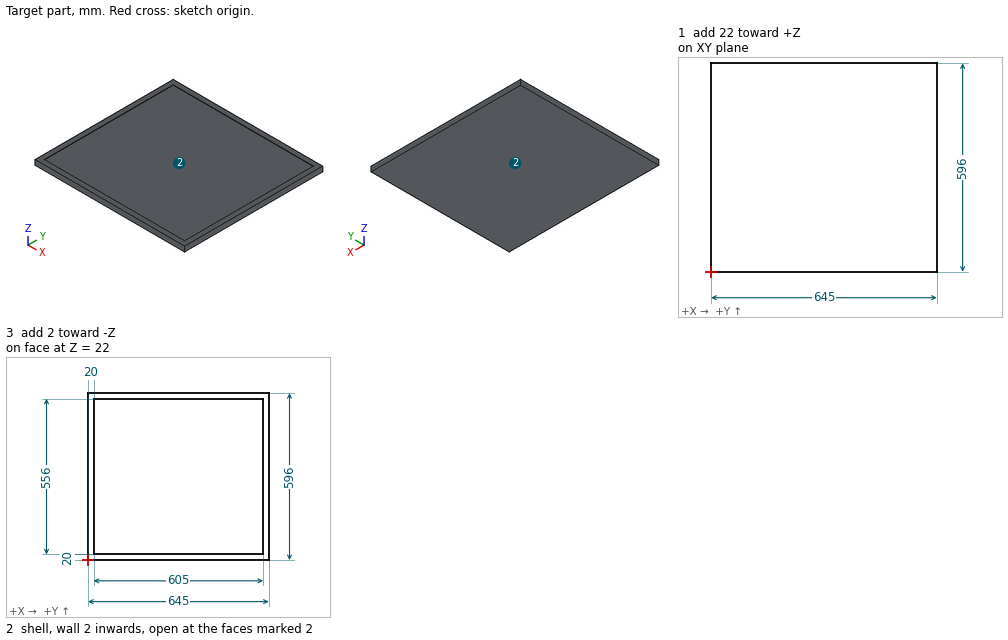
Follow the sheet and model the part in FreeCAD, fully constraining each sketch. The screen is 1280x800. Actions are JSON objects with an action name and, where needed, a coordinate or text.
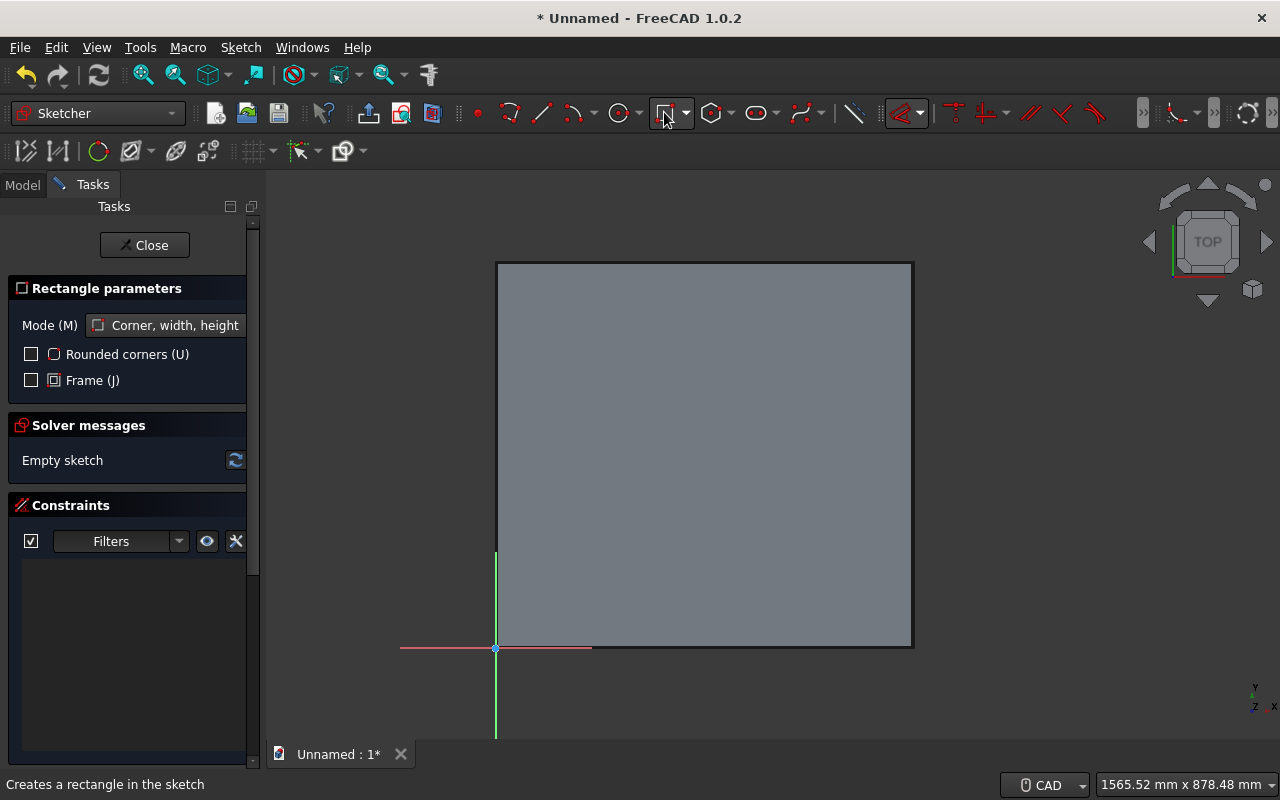
{"action": "left_click", "coordinate": [496, 648]}
{"action": "left_click", "coordinate": [914, 262]}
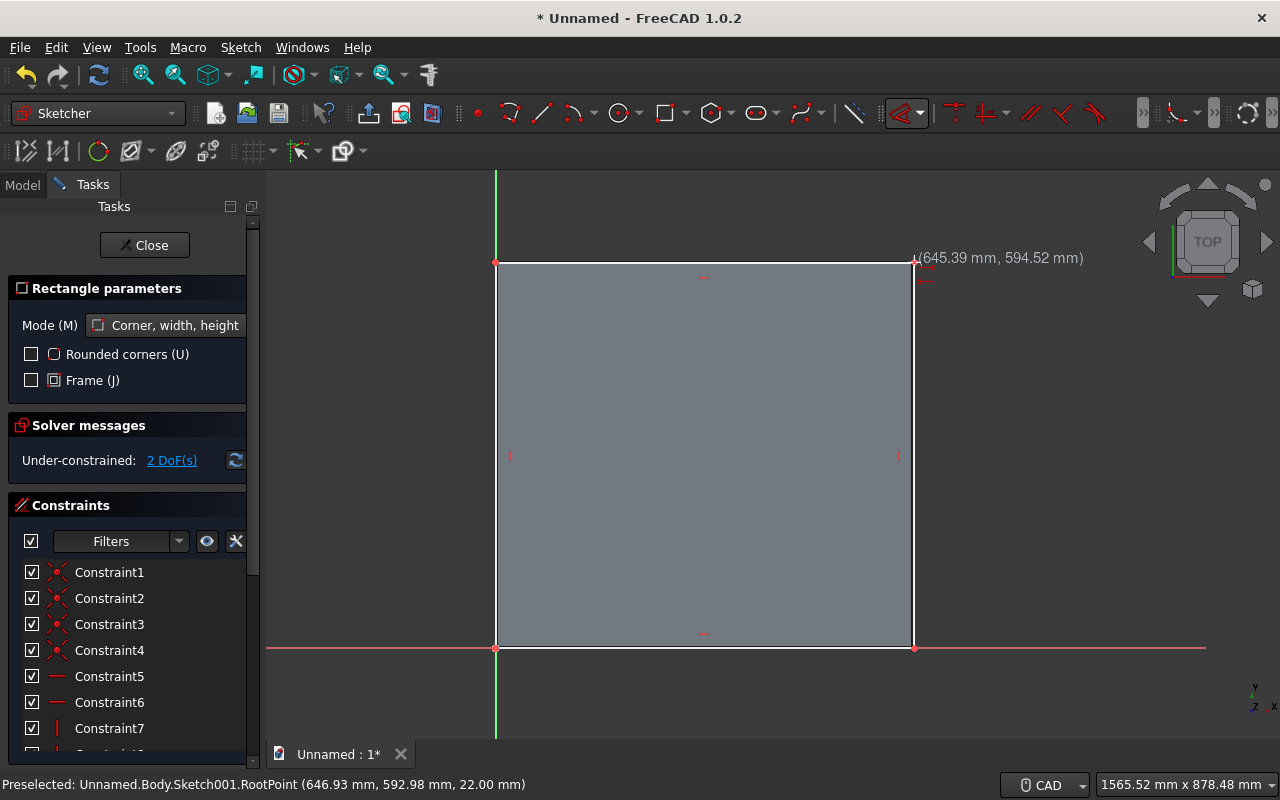
{"action": "scroll", "coordinate": [509, 275], "scroll_direction": "up", "scroll_amount": 2}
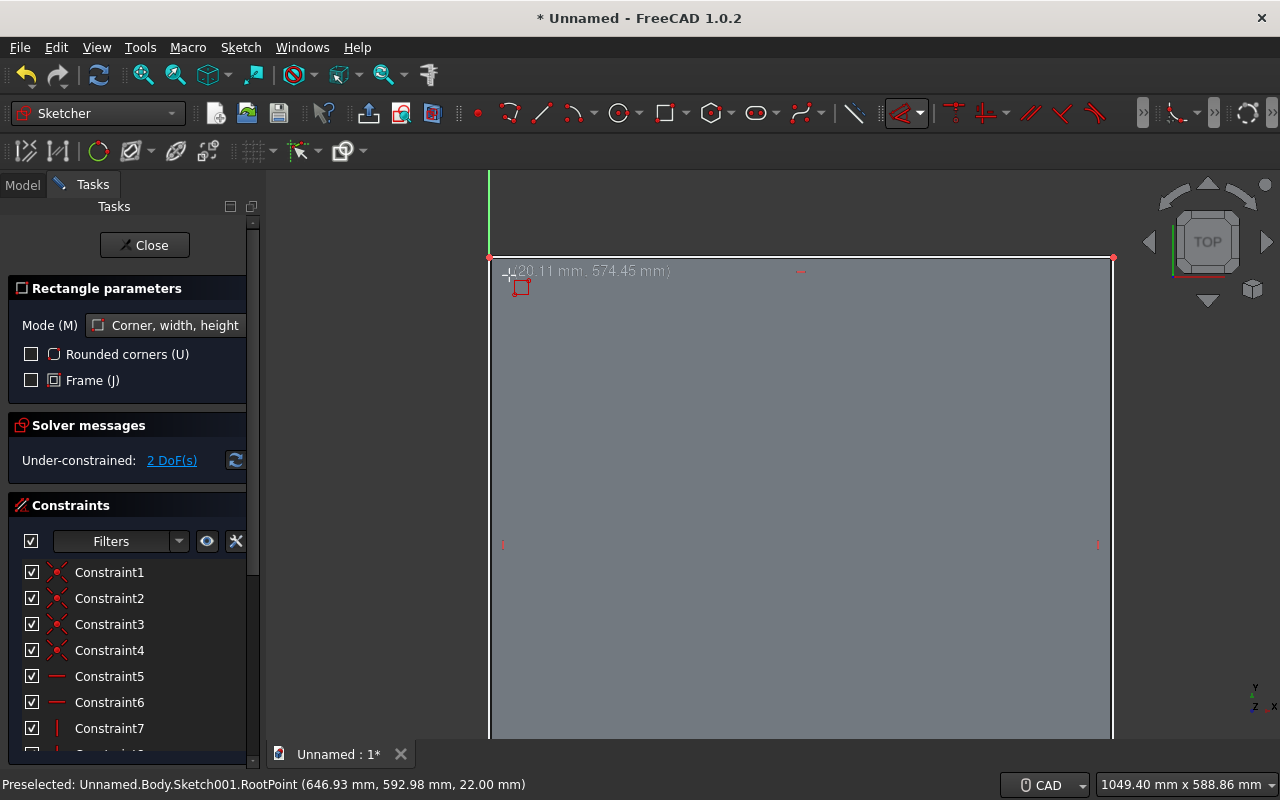
{"action": "left_click", "coordinate": [509, 275]}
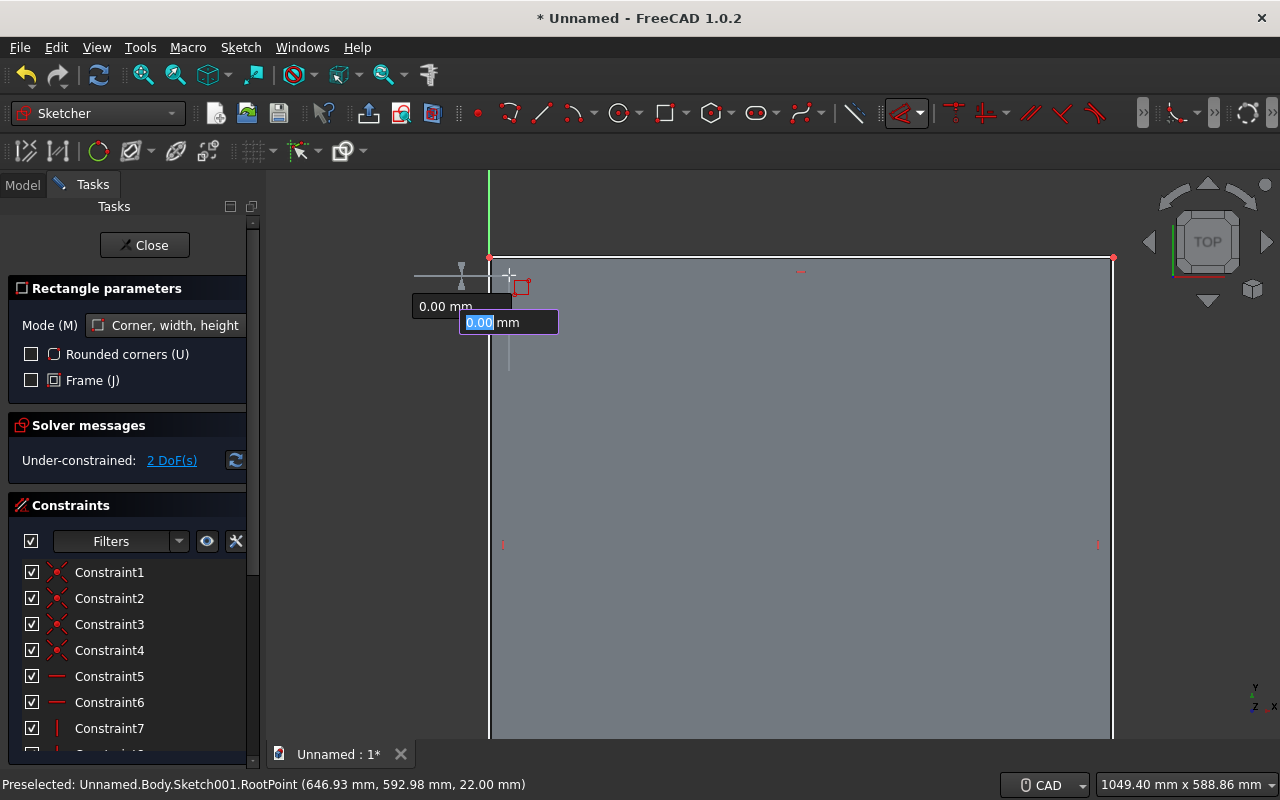
{"action": "scroll", "coordinate": [508, 273], "scroll_direction": "down", "scroll_amount": 2}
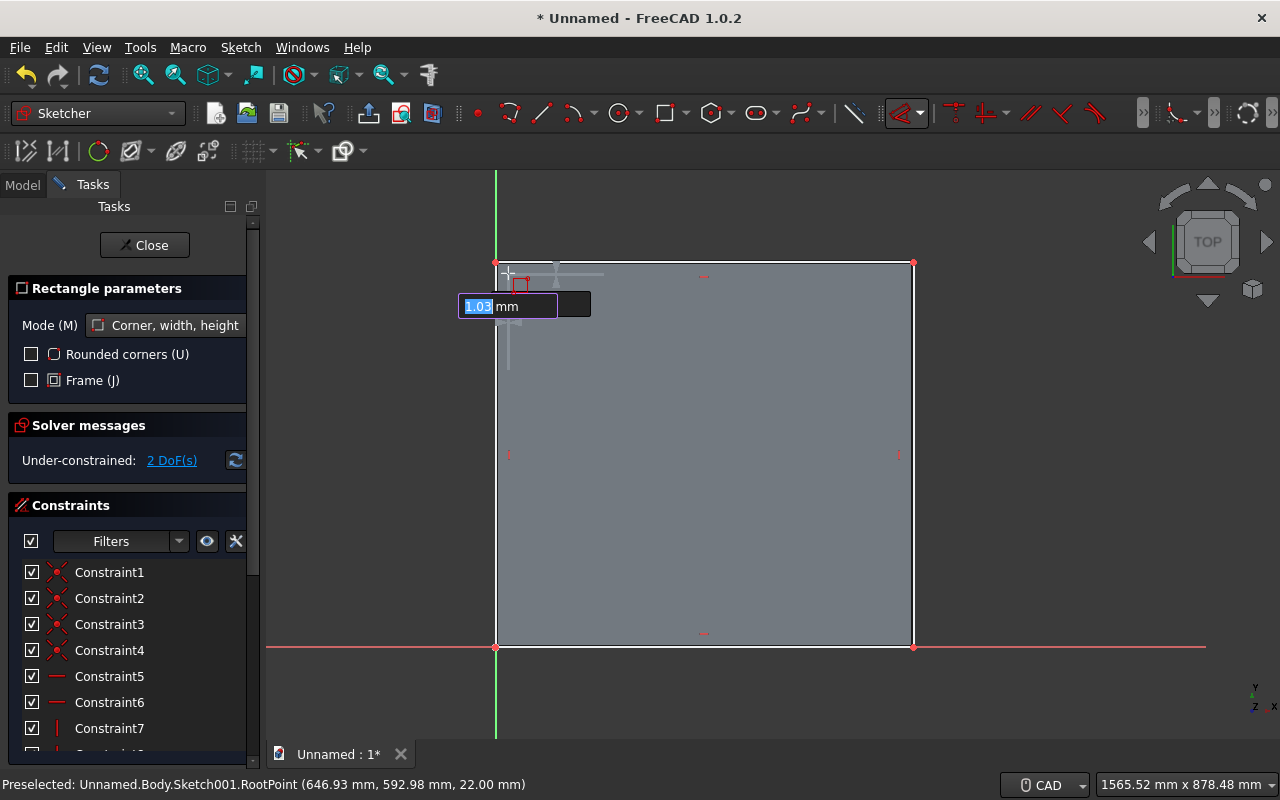
{"action": "scroll", "coordinate": [900, 634], "scroll_direction": "up", "scroll_amount": 2}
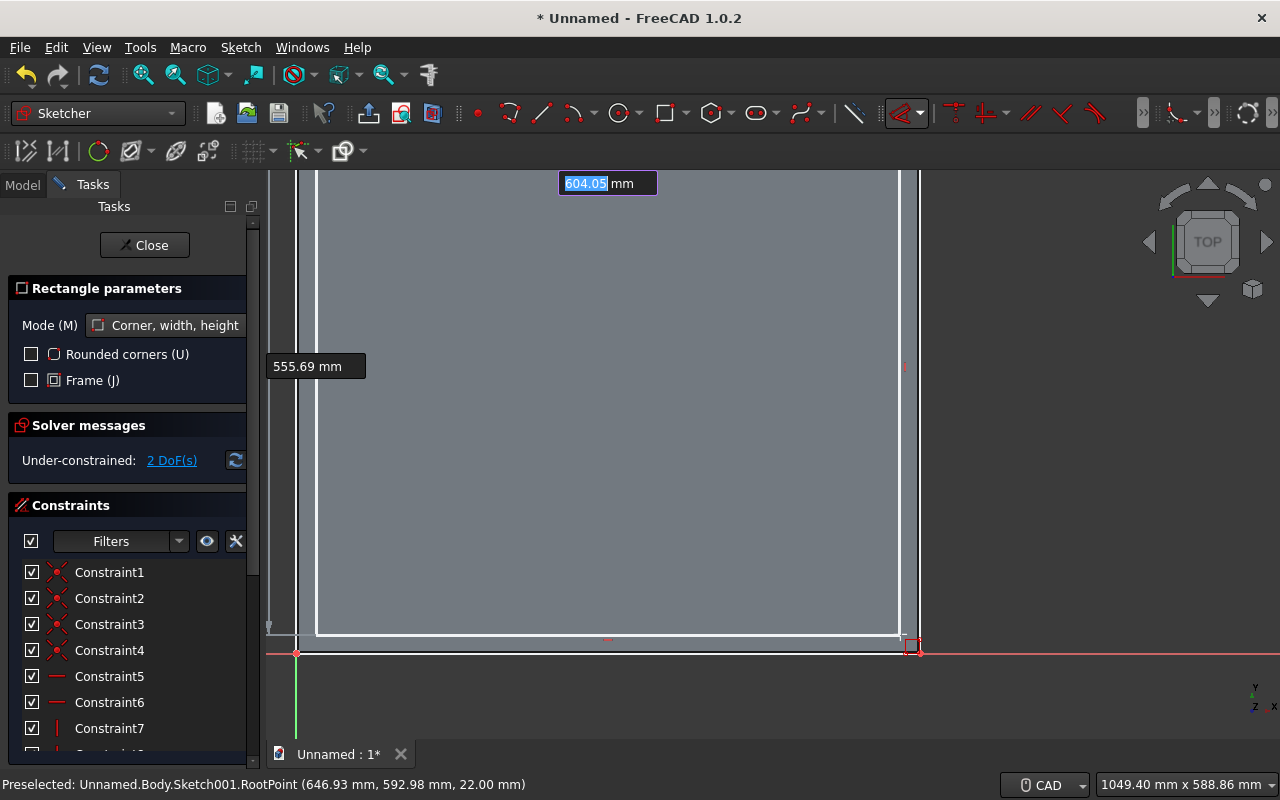
{"action": "left_click", "coordinate": [900, 634]}
{"action": "key", "text": "Escape"}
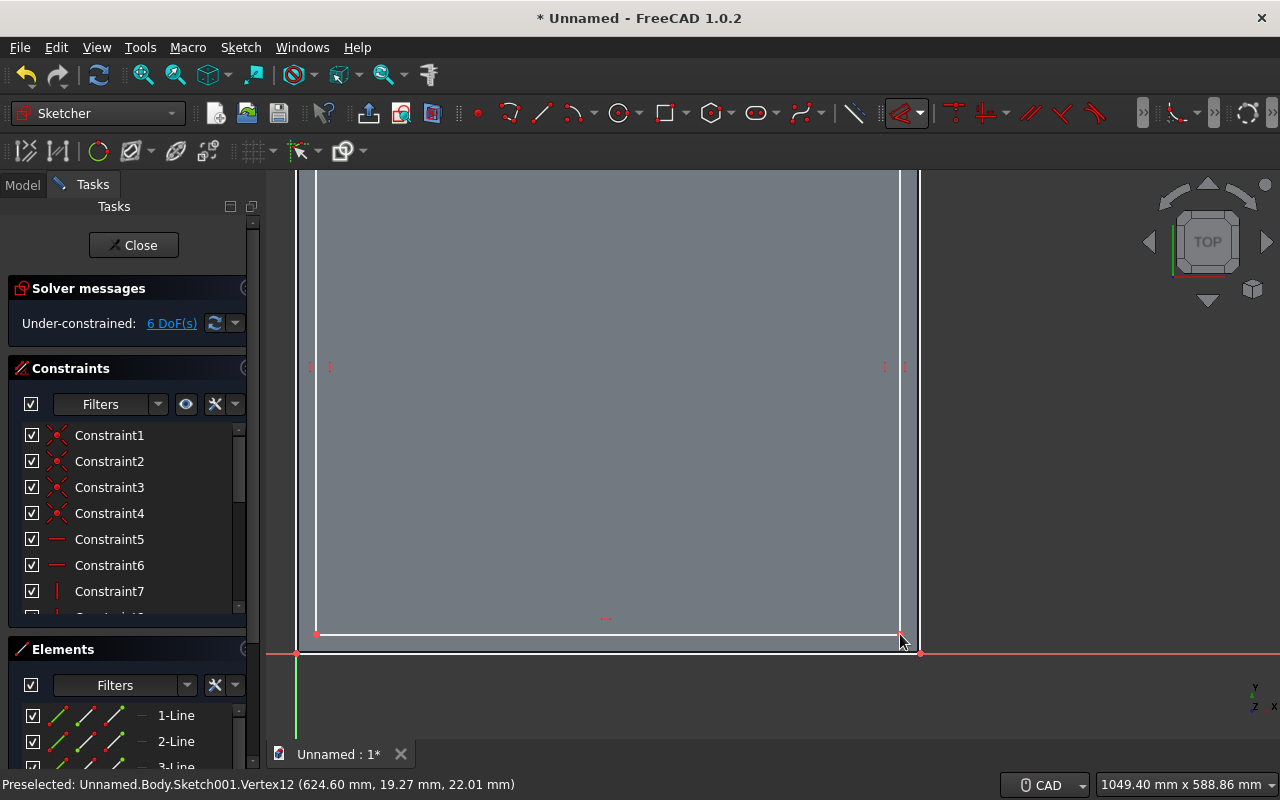
{"action": "left_click", "coordinate": [484, 654]}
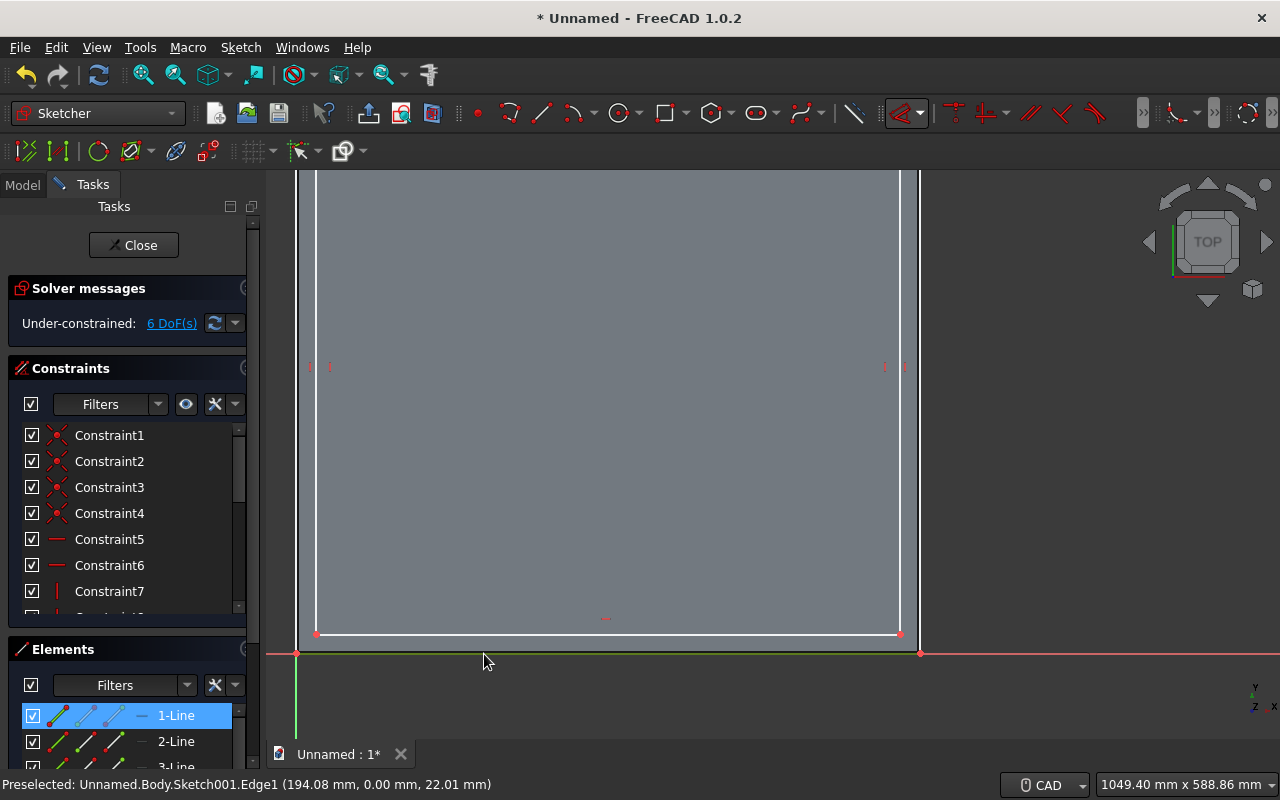
{"action": "left_click", "coordinate": [922, 114]}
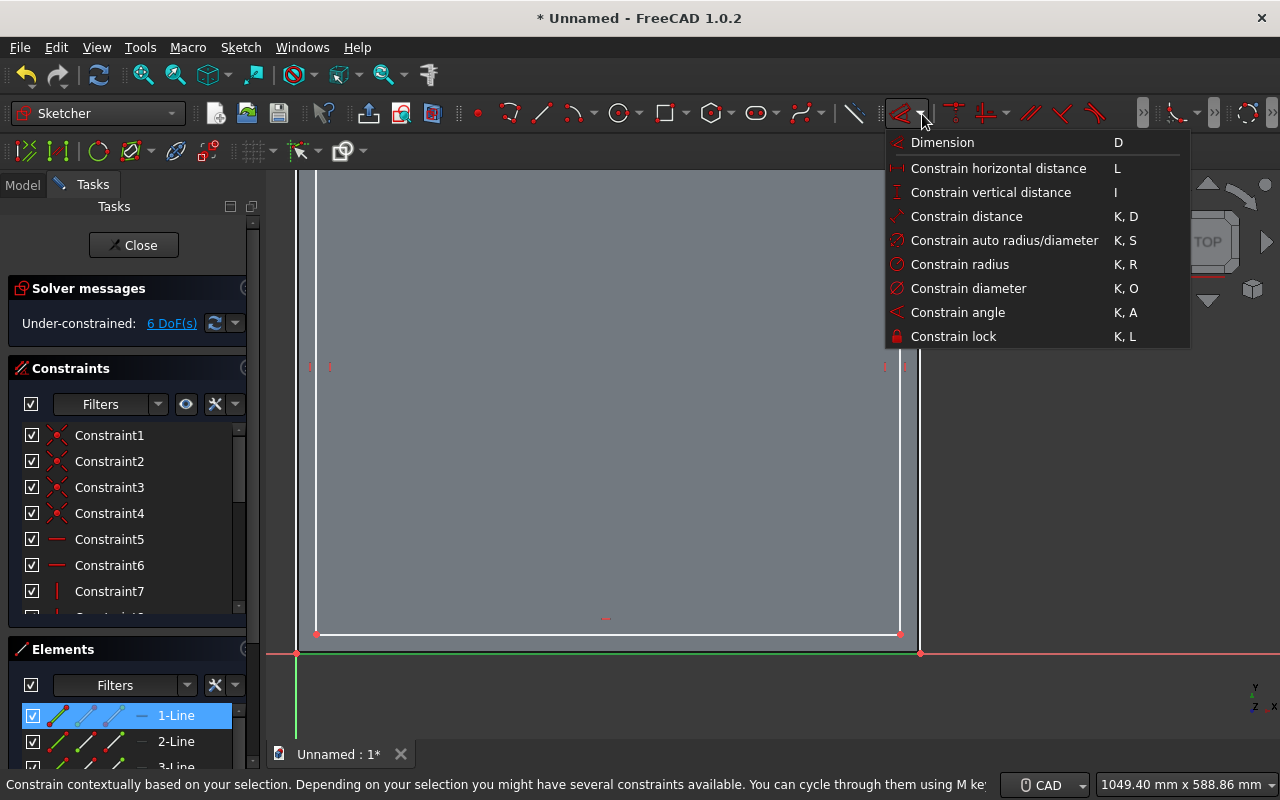
{"action": "left_click", "coordinate": [1038, 168]}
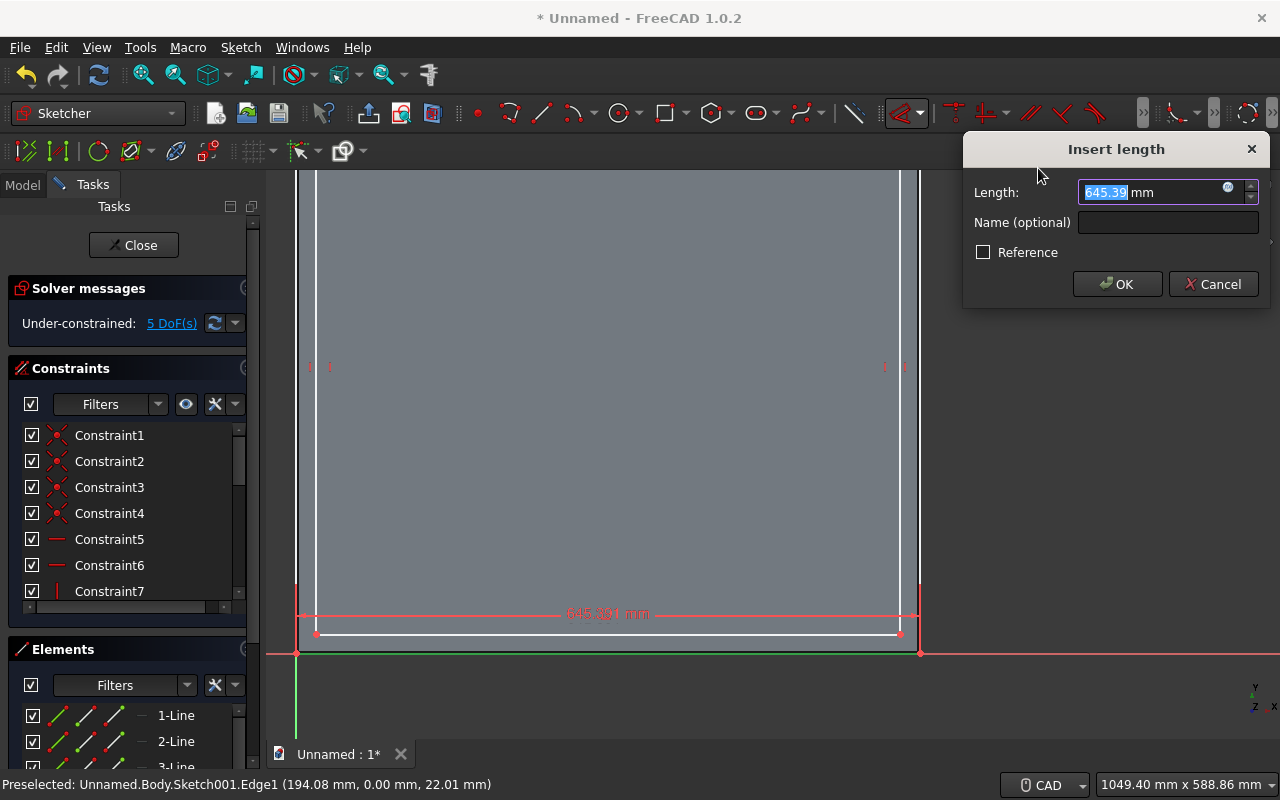
{"action": "type", "text": "645"}
{"action": "key", "text": "Return"}